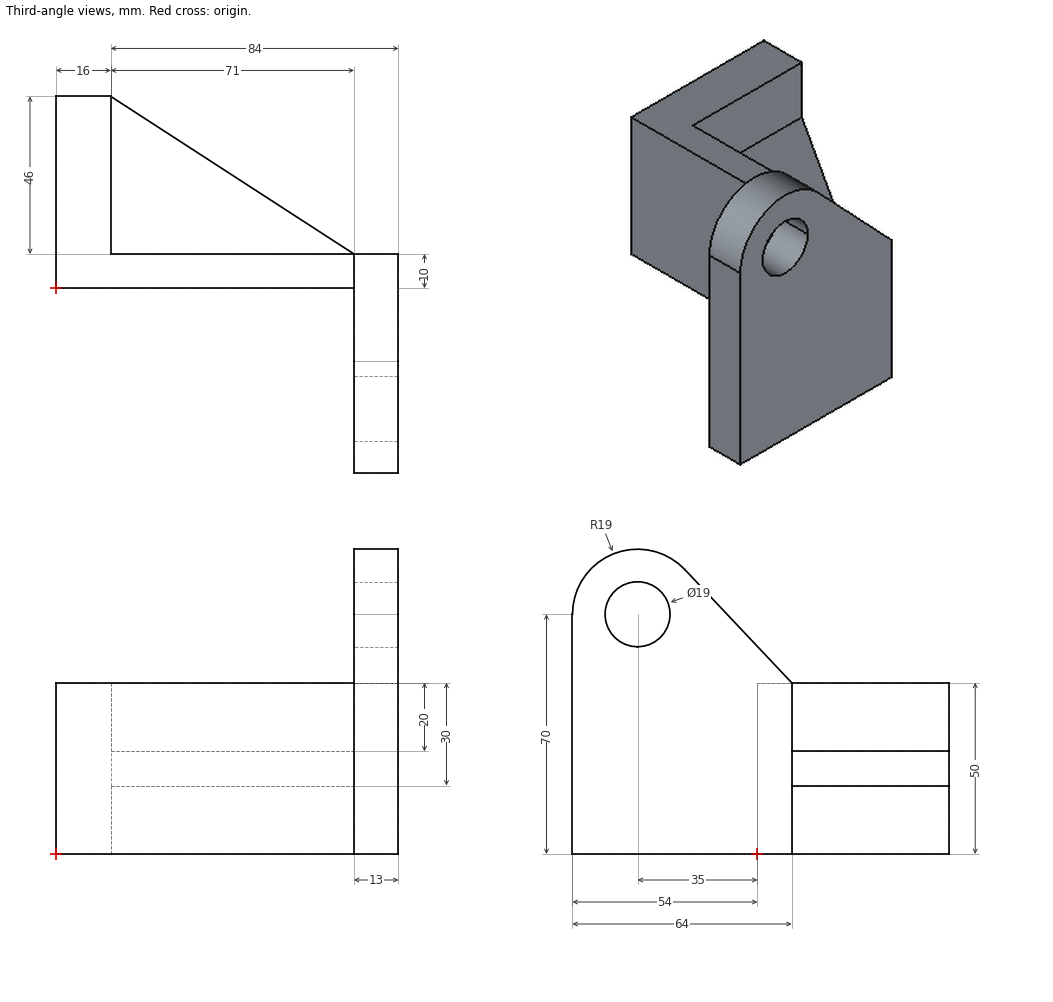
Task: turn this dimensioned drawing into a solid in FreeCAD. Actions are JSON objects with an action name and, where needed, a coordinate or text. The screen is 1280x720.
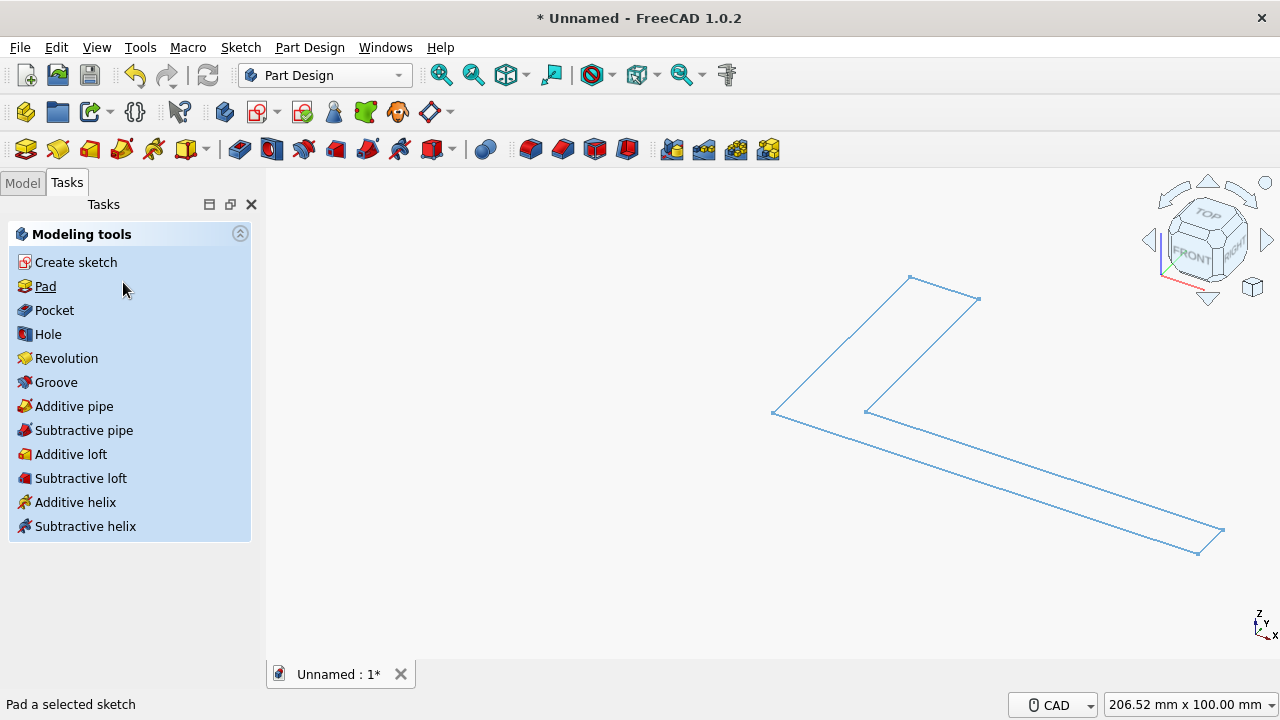
{"action": "left_click", "coordinate": [26, 150]}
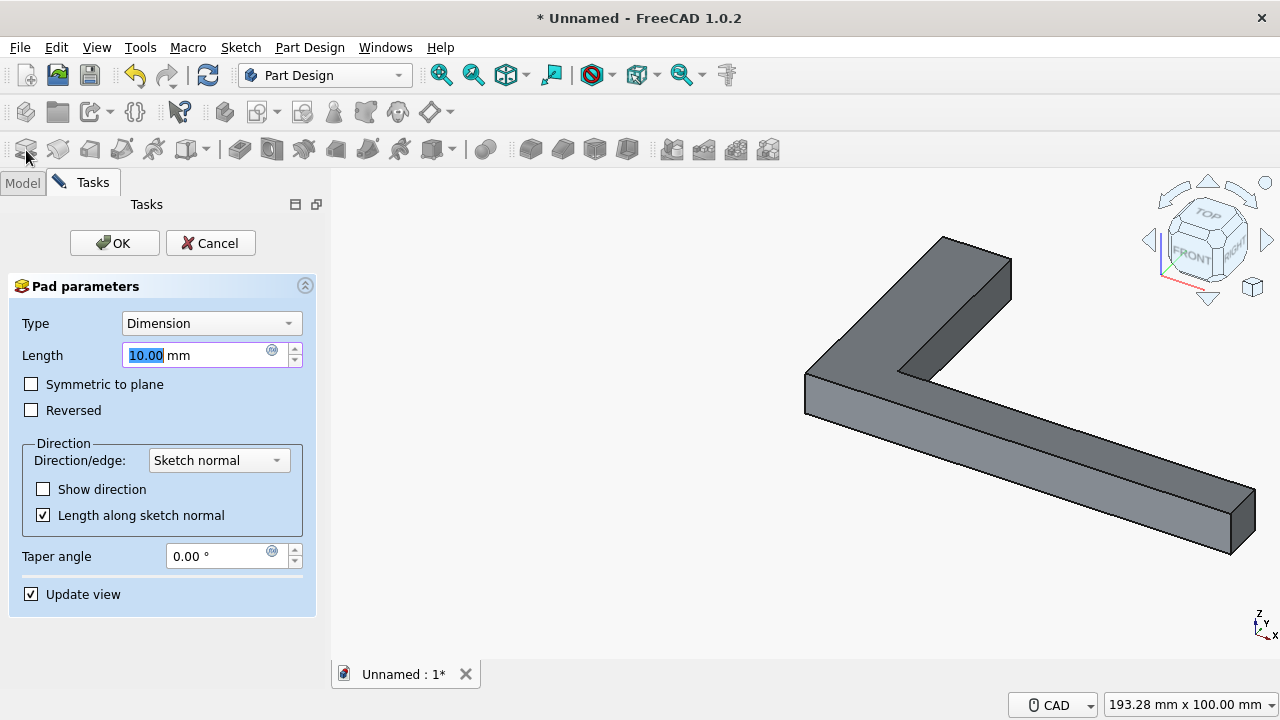
{"action": "type", "text": "50"}
{"action": "key", "text": "Tab"}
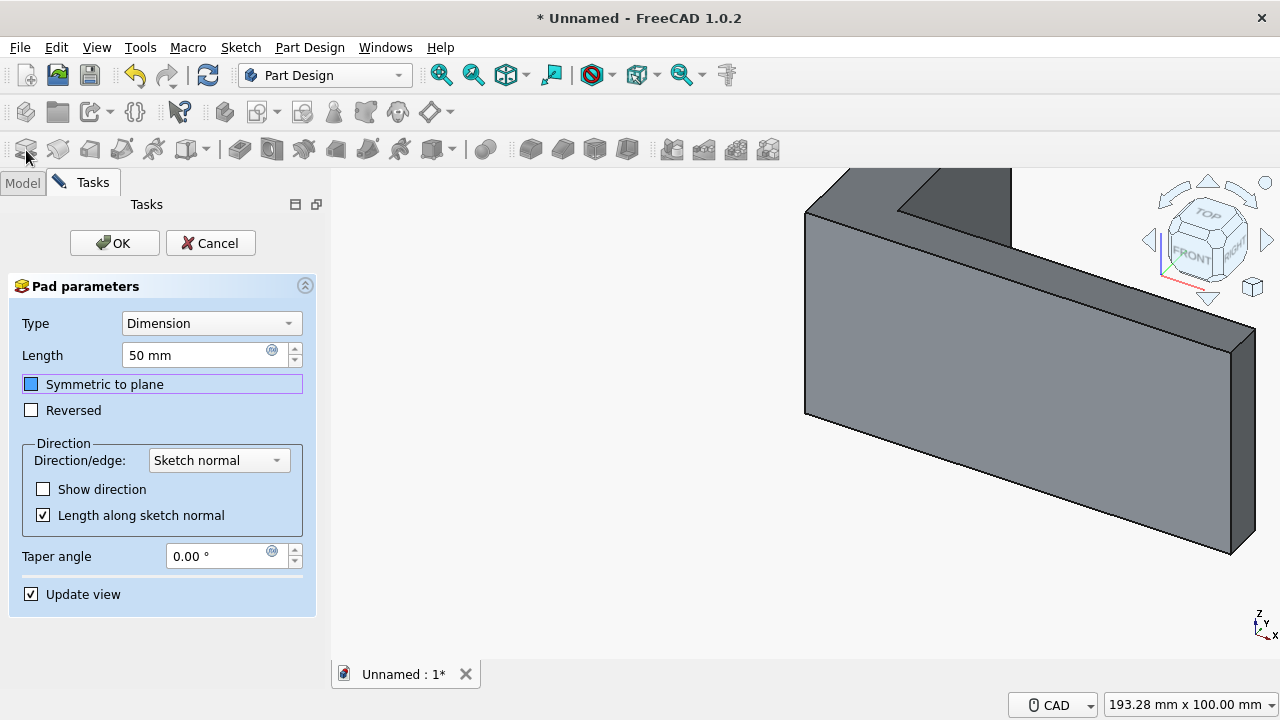
{"action": "left_click", "coordinate": [115, 243]}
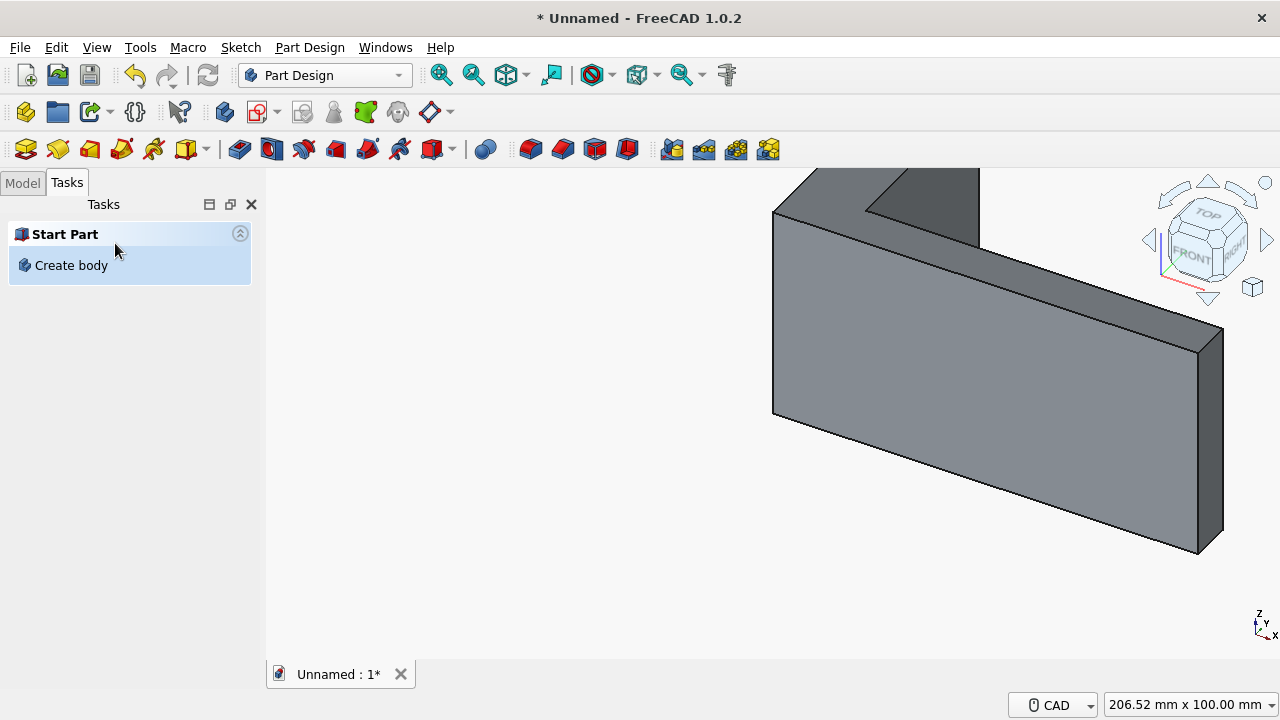
{"action": "left_click", "coordinate": [442, 76]}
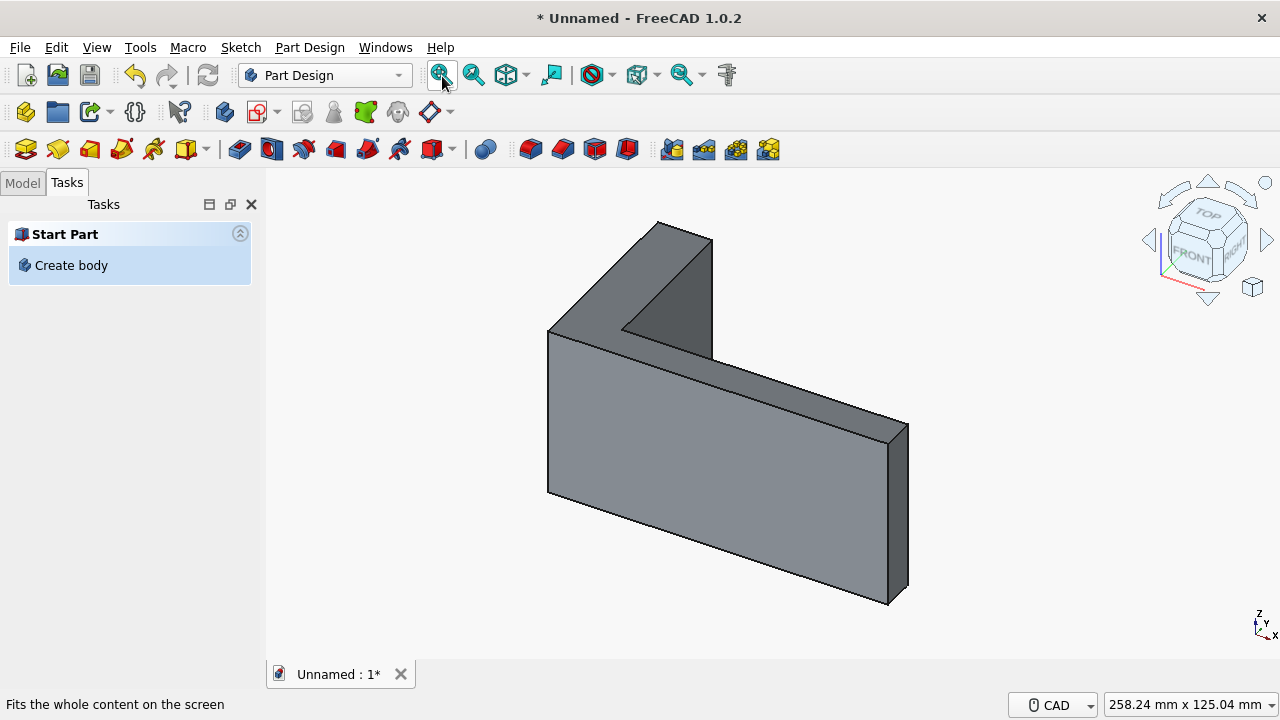
{"action": "left_click", "coordinate": [898, 468]}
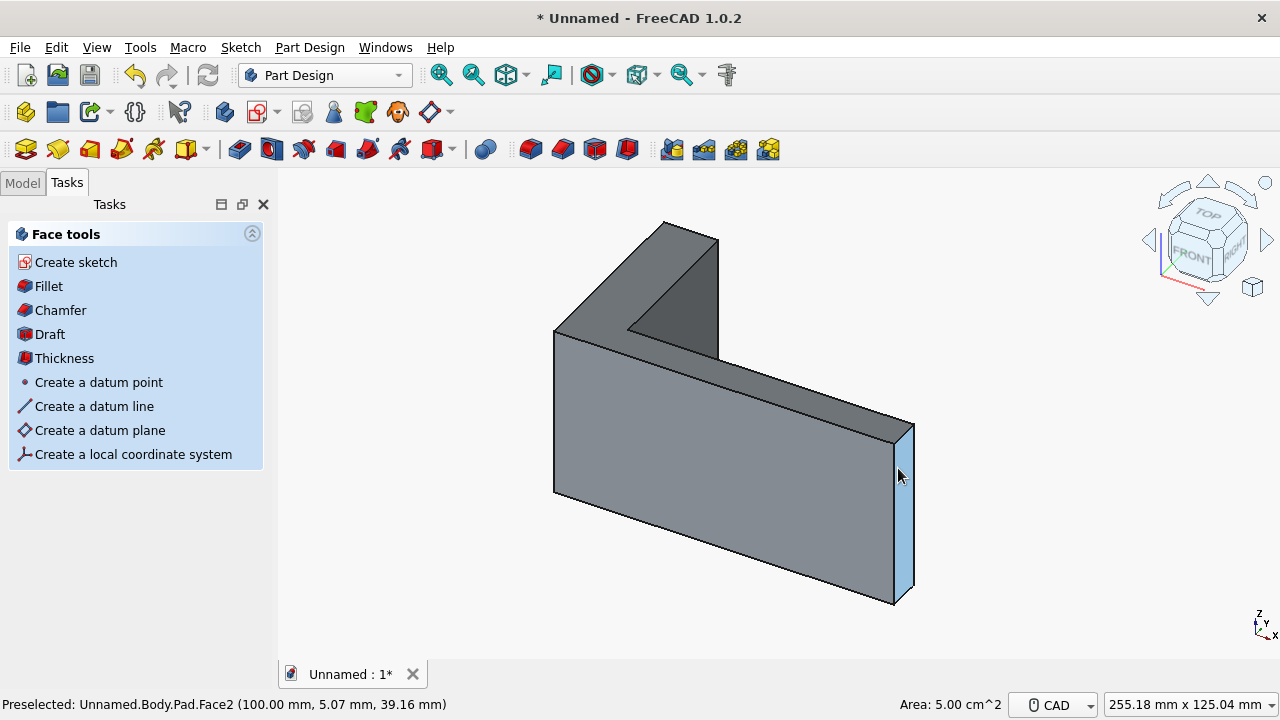
{"action": "left_click", "coordinate": [258, 112]}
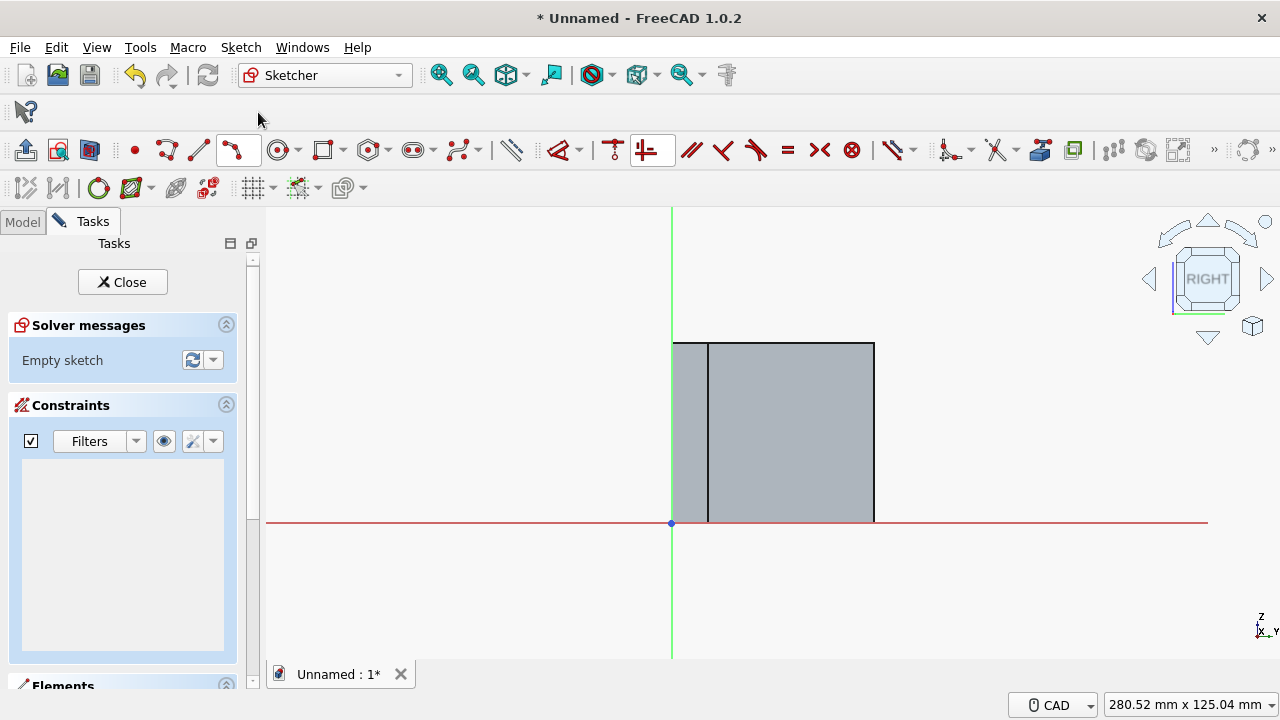
{"action": "scroll", "coordinate": [1115, 631], "scroll_direction": "down", "scroll_amount": 1}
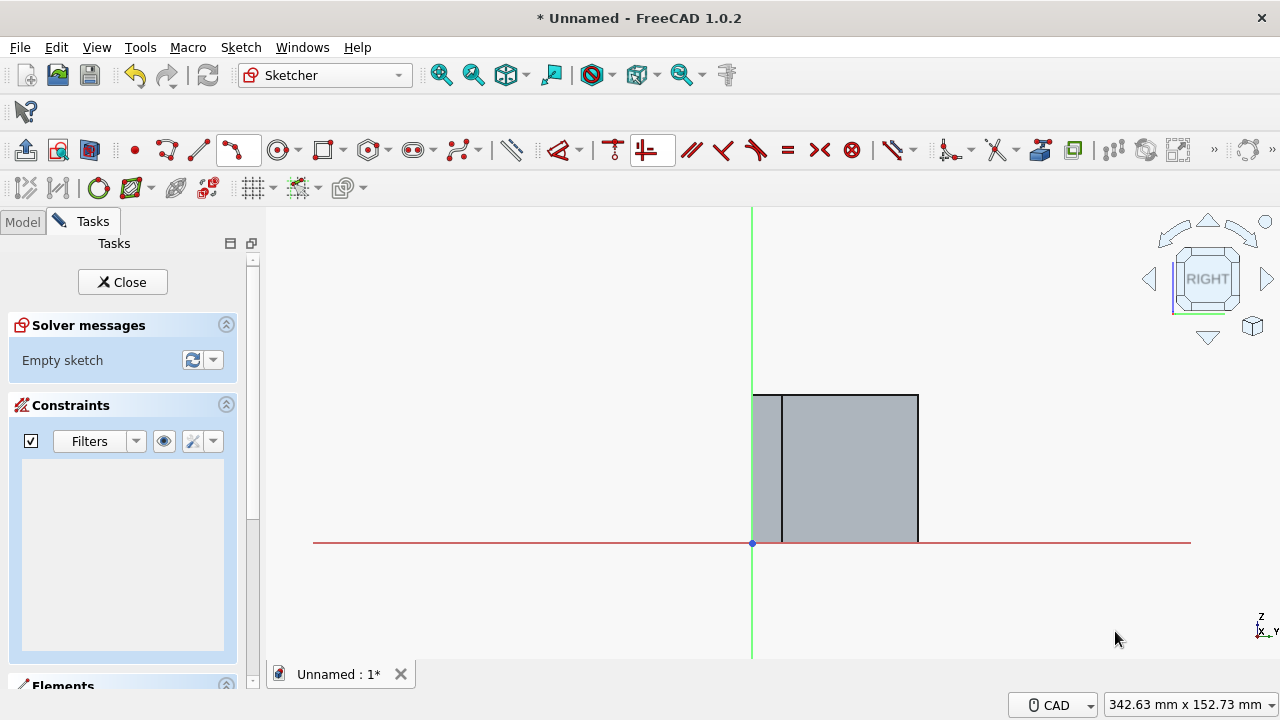
{"action": "key", "text": "g m"}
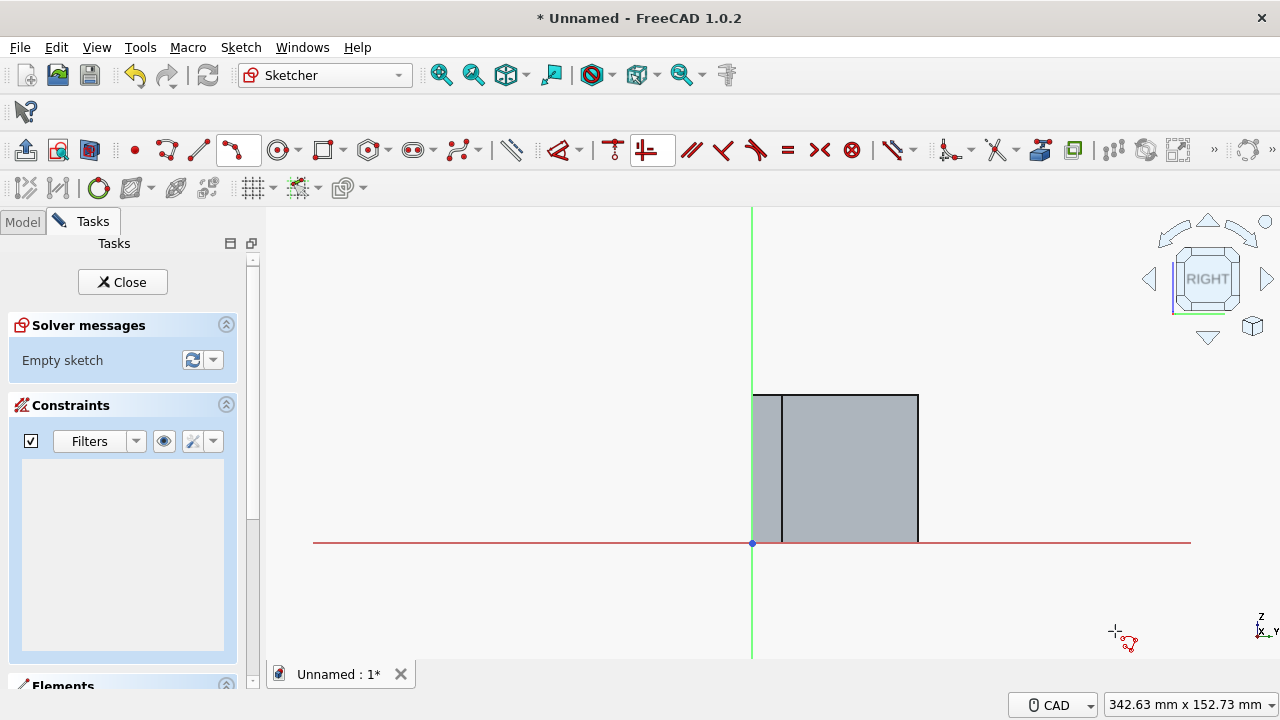
{"action": "left_click", "coordinate": [592, 336]}
{"action": "left_click", "coordinate": [592, 543]}
{"action": "left_click", "coordinate": [782, 534]}
{"action": "left_click", "coordinate": [782, 395]}
{"action": "left_click", "coordinate": [690, 297]}
{"action": "right_click", "coordinate": [690, 297]}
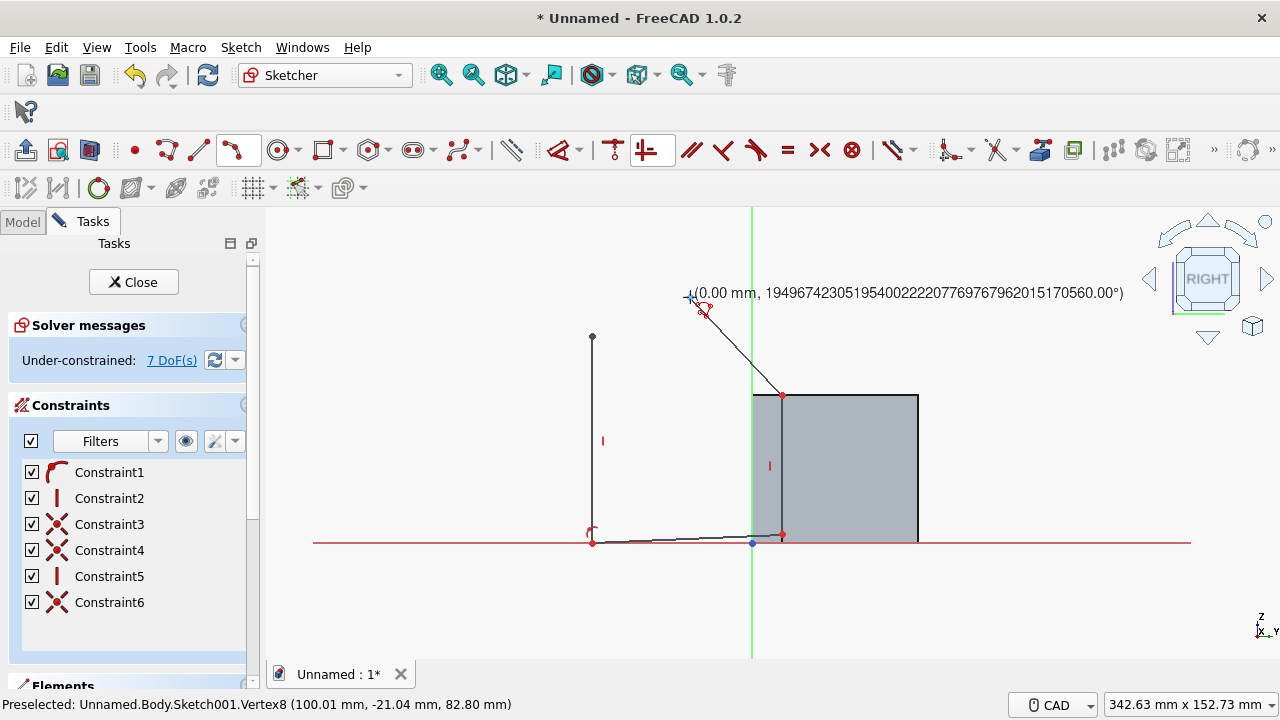
{"action": "key", "text": "g 3 a"}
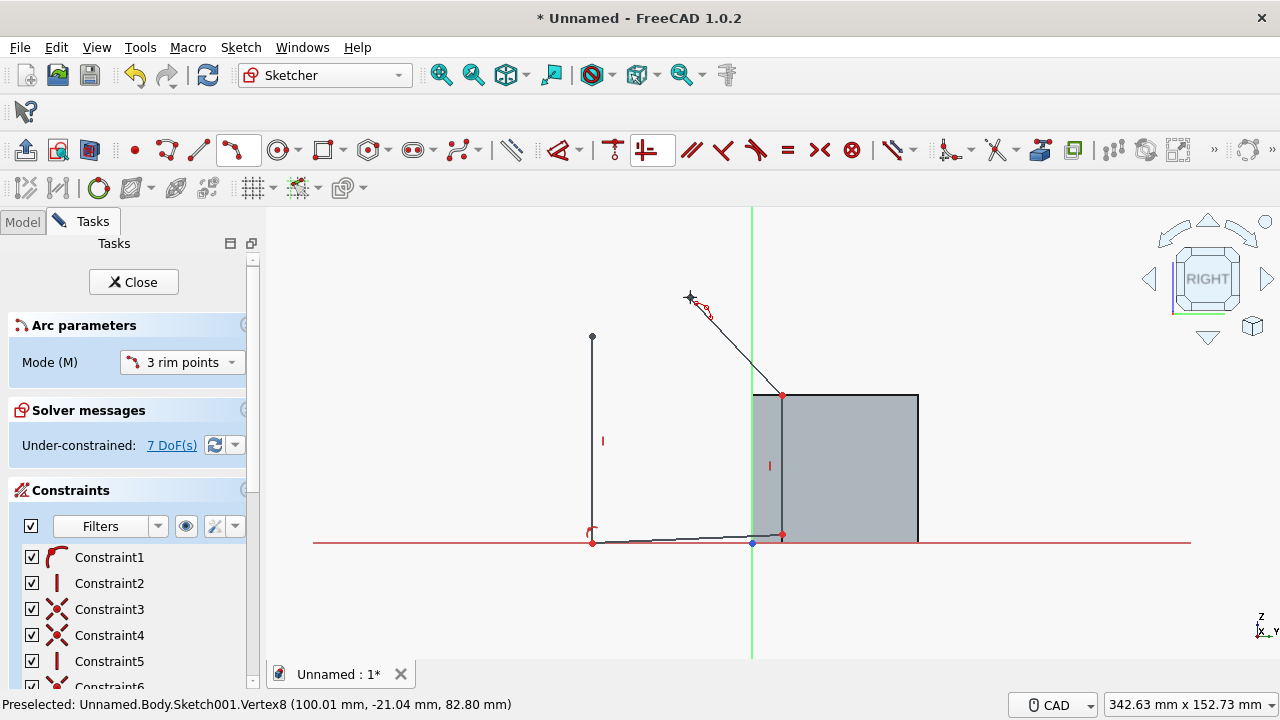
{"action": "left_click", "coordinate": [690, 298]}
{"action": "left_click", "coordinate": [592, 337]}
{"action": "left_click", "coordinate": [628, 284]}
{"action": "key", "text": "Escape"}